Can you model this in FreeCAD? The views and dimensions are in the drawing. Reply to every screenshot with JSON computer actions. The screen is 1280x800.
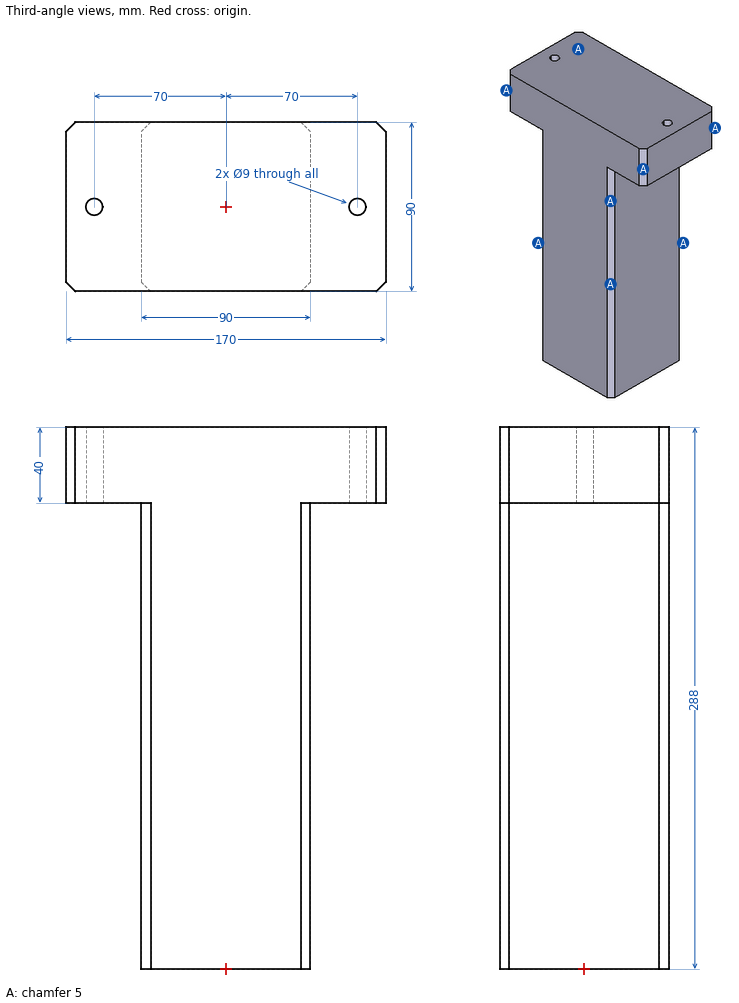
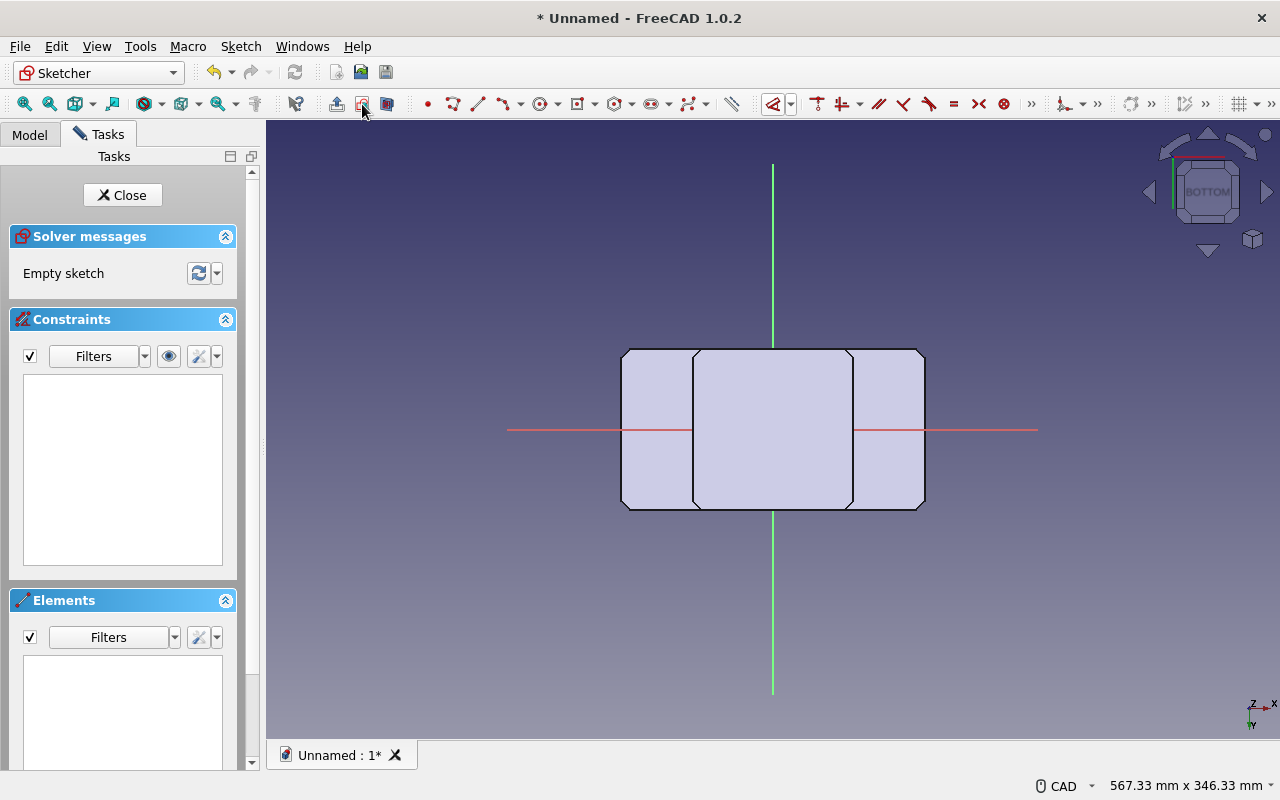
{"action": "scroll", "coordinate": [829, 430], "scroll_direction": "up", "scroll_amount": 4}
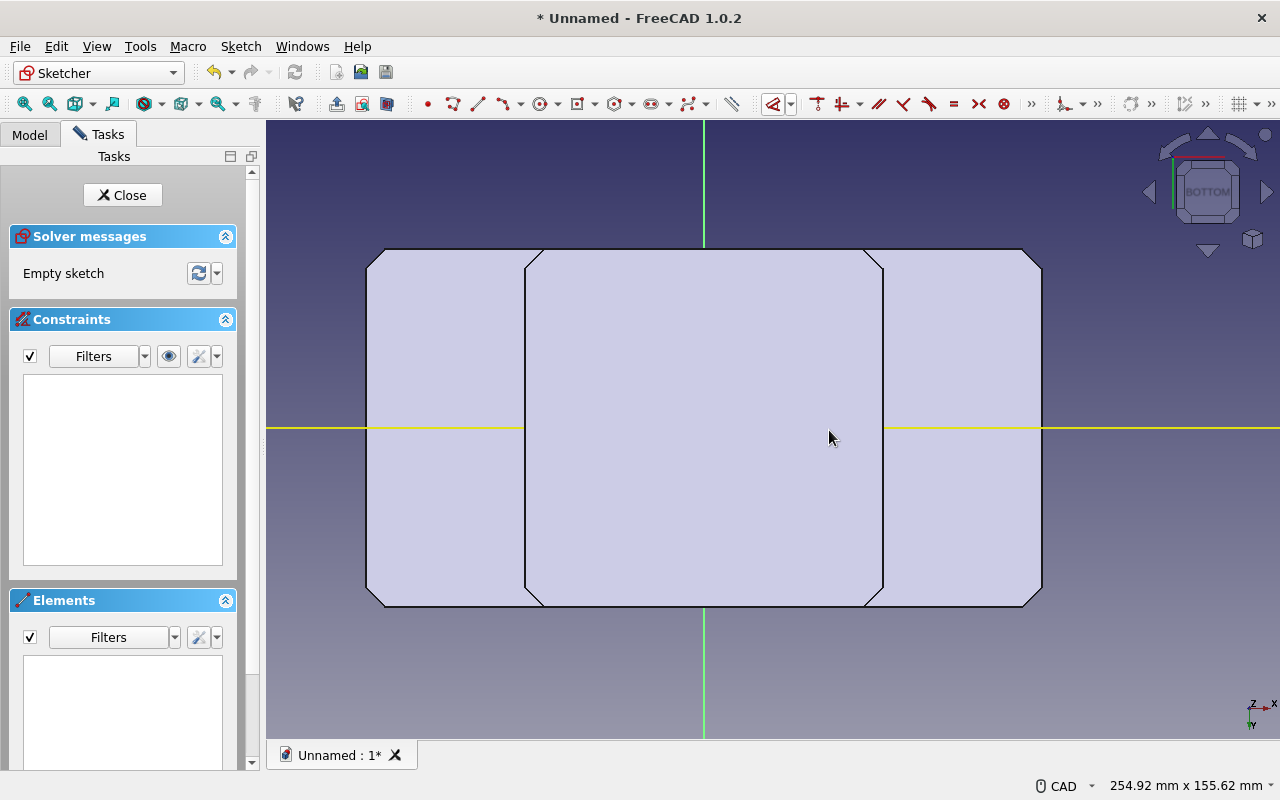
{"action": "left_click", "coordinate": [540, 104]}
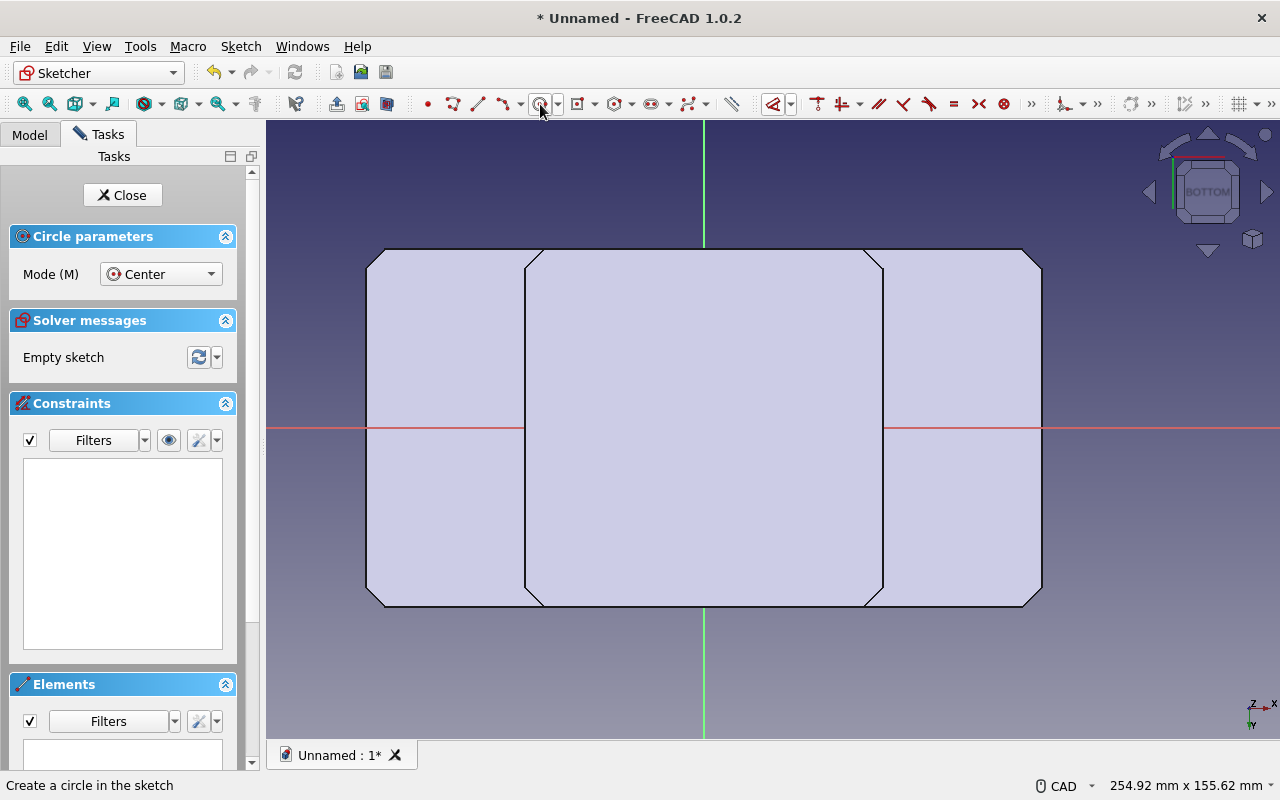
{"action": "scroll", "coordinate": [982, 428], "scroll_direction": "up", "scroll_amount": 2}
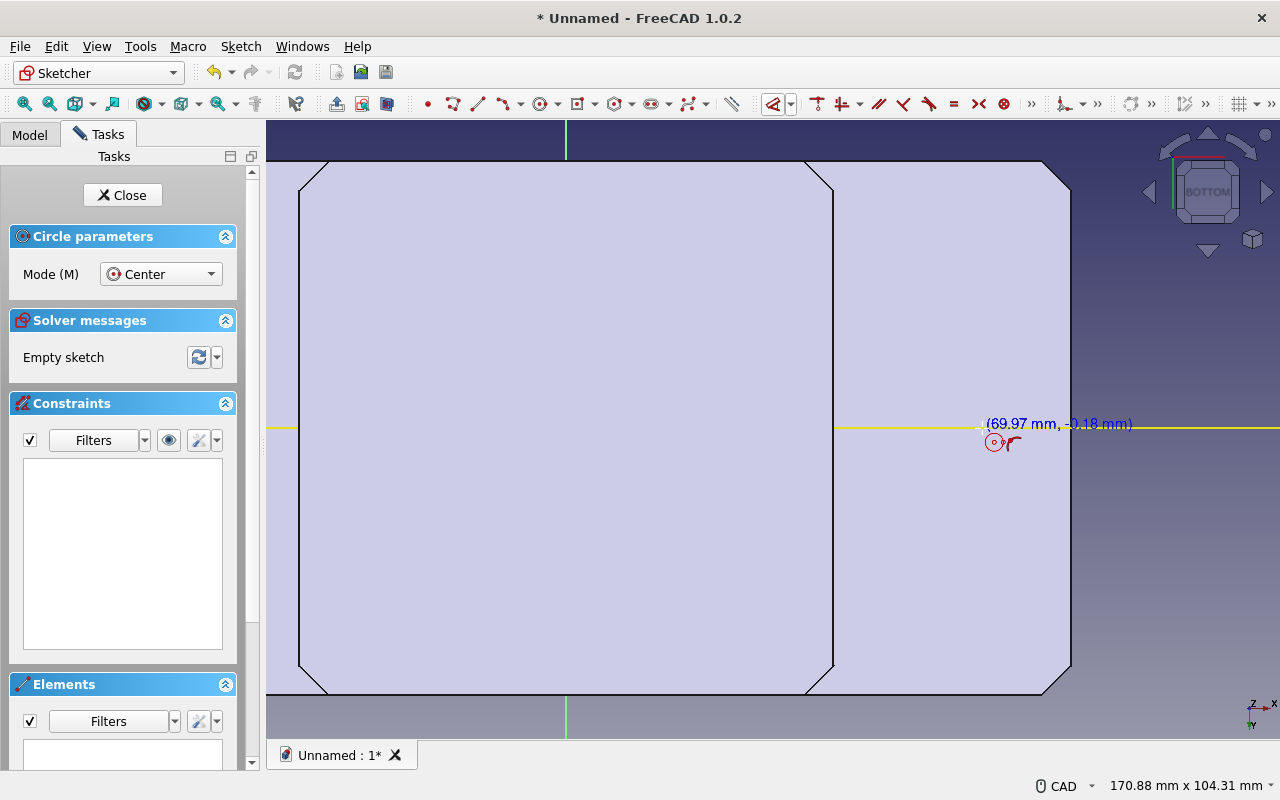
{"action": "left_click", "coordinate": [982, 428]}
{"action": "left_click", "coordinate": [1001, 409]}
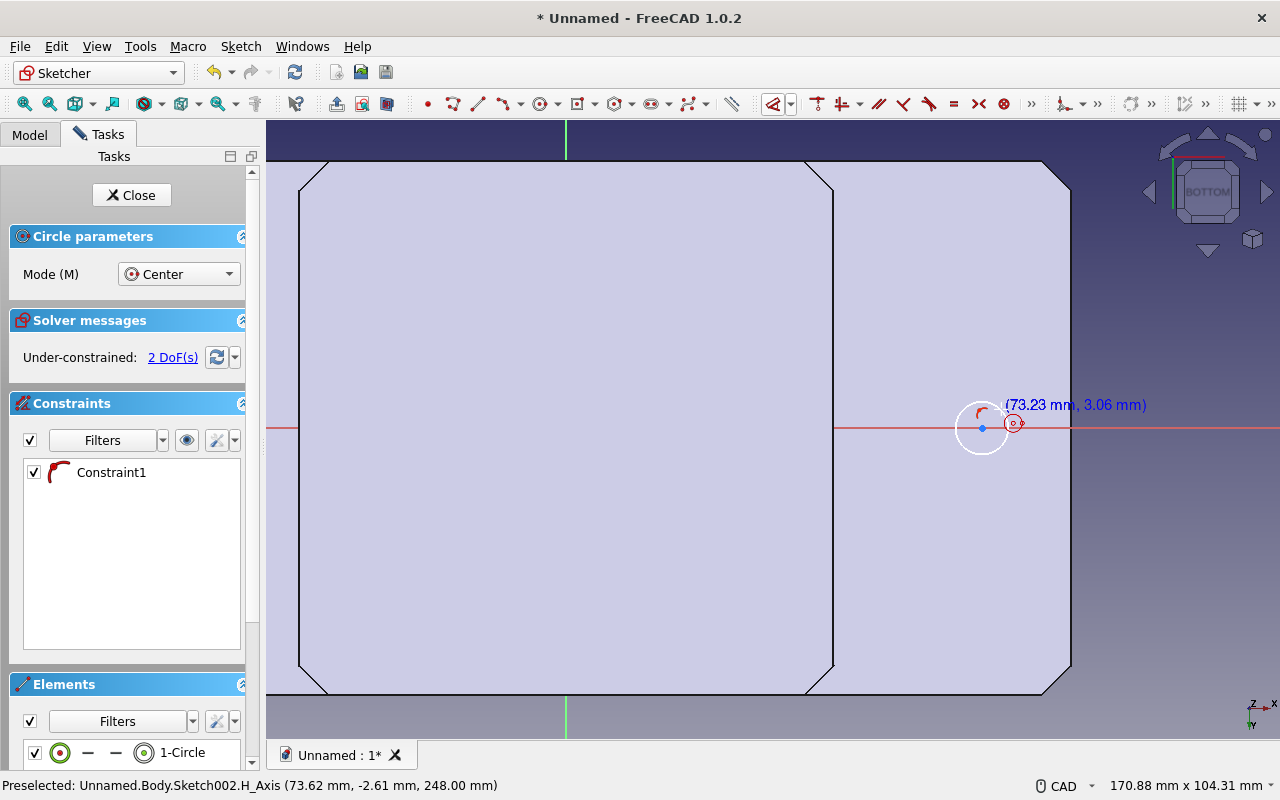
{"action": "scroll", "coordinate": [985, 432], "scroll_direction": "down", "scroll_amount": 2}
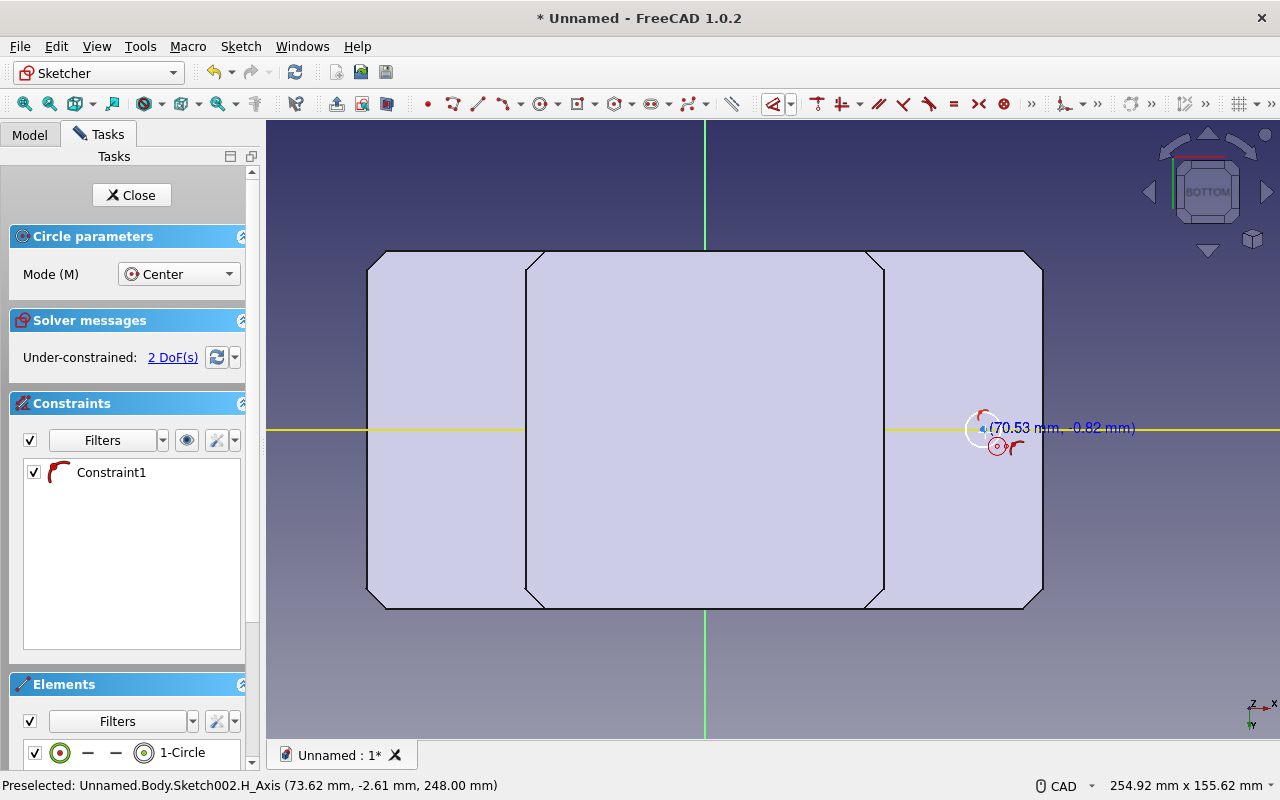
{"action": "scroll", "coordinate": [426, 430], "scroll_direction": "up", "scroll_amount": 2}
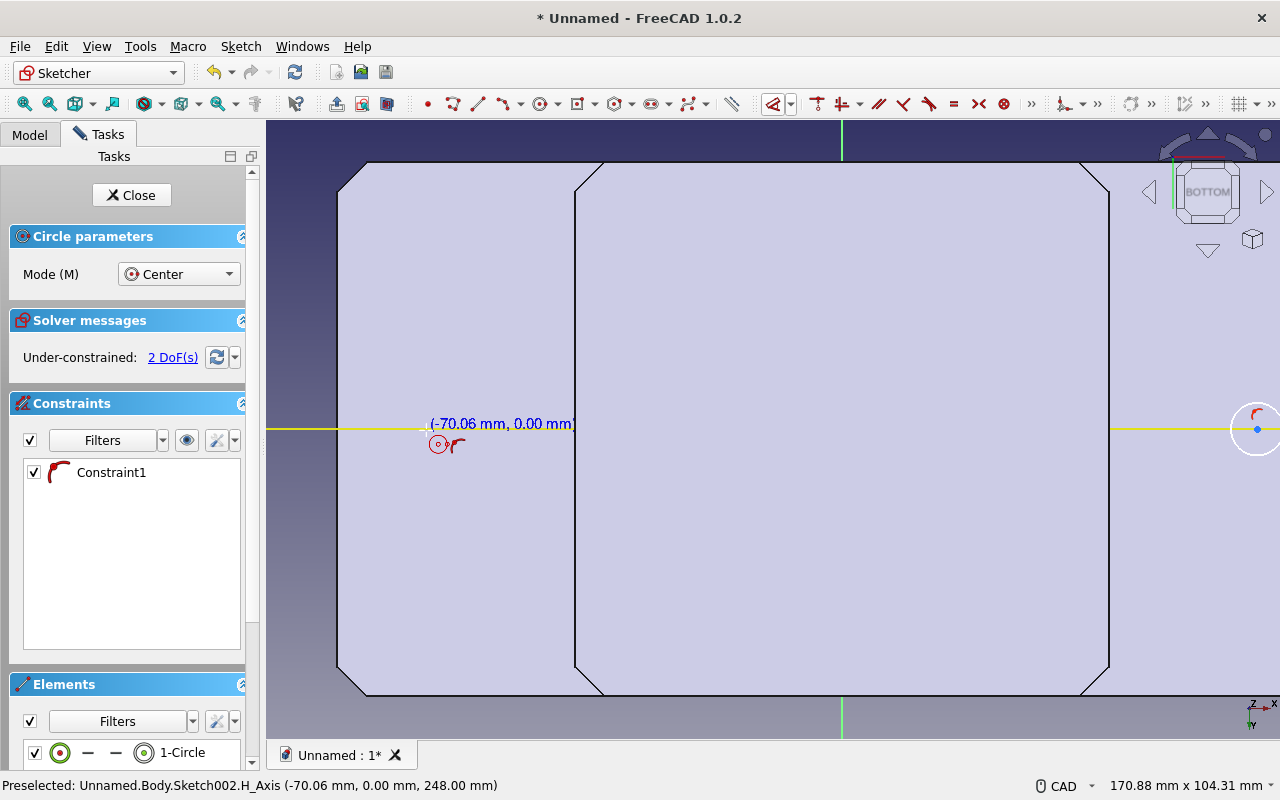
{"action": "left_click", "coordinate": [426, 429]}
{"action": "left_click", "coordinate": [445, 410]}
{"action": "key", "text": "Escape"}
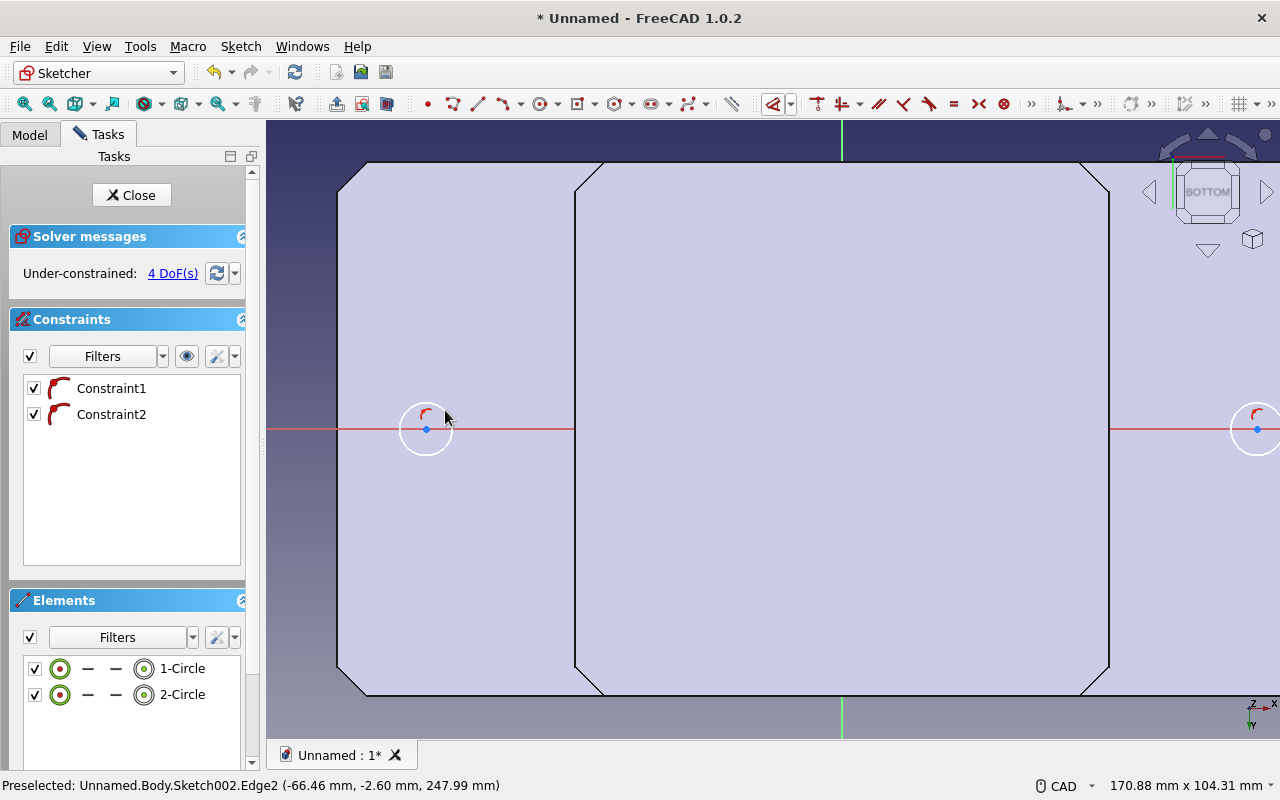
{"action": "scroll", "coordinate": [426, 430], "scroll_direction": "down", "scroll_amount": 2}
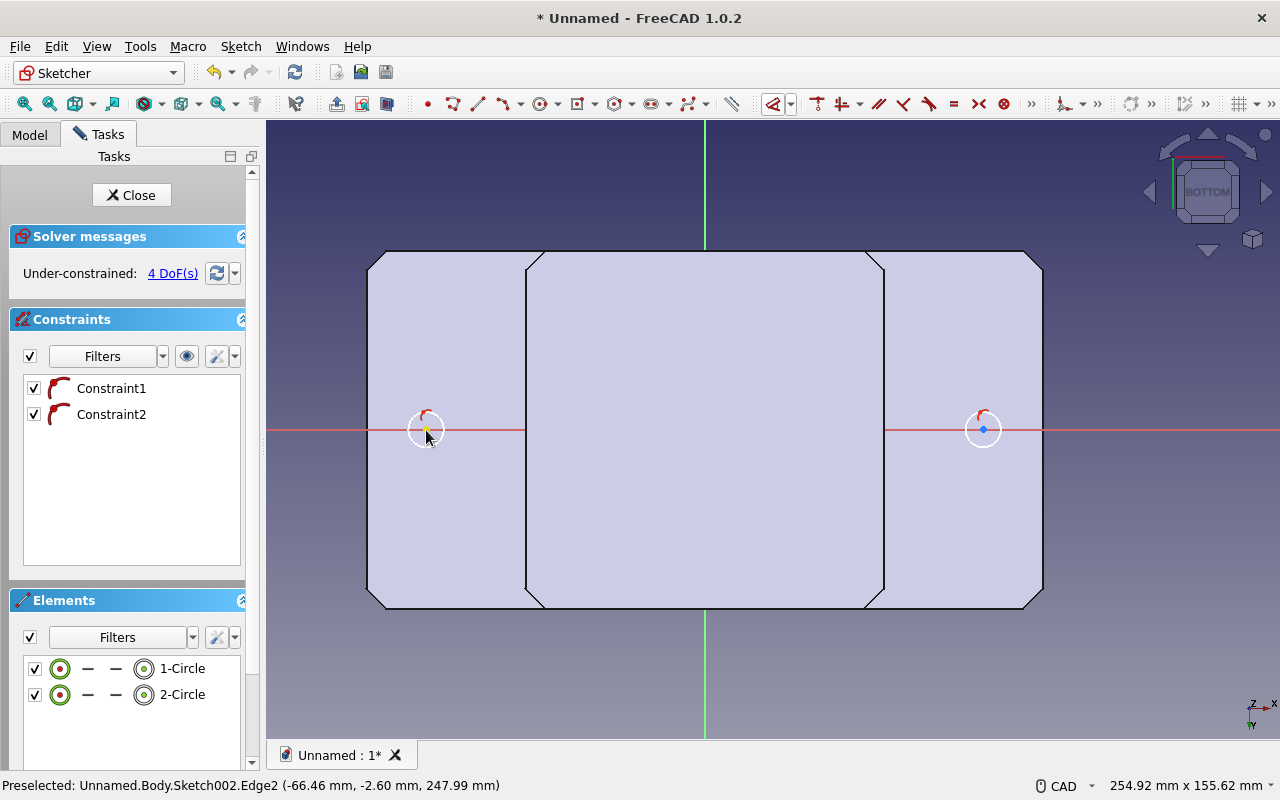
{"action": "left_click", "coordinate": [996, 417]}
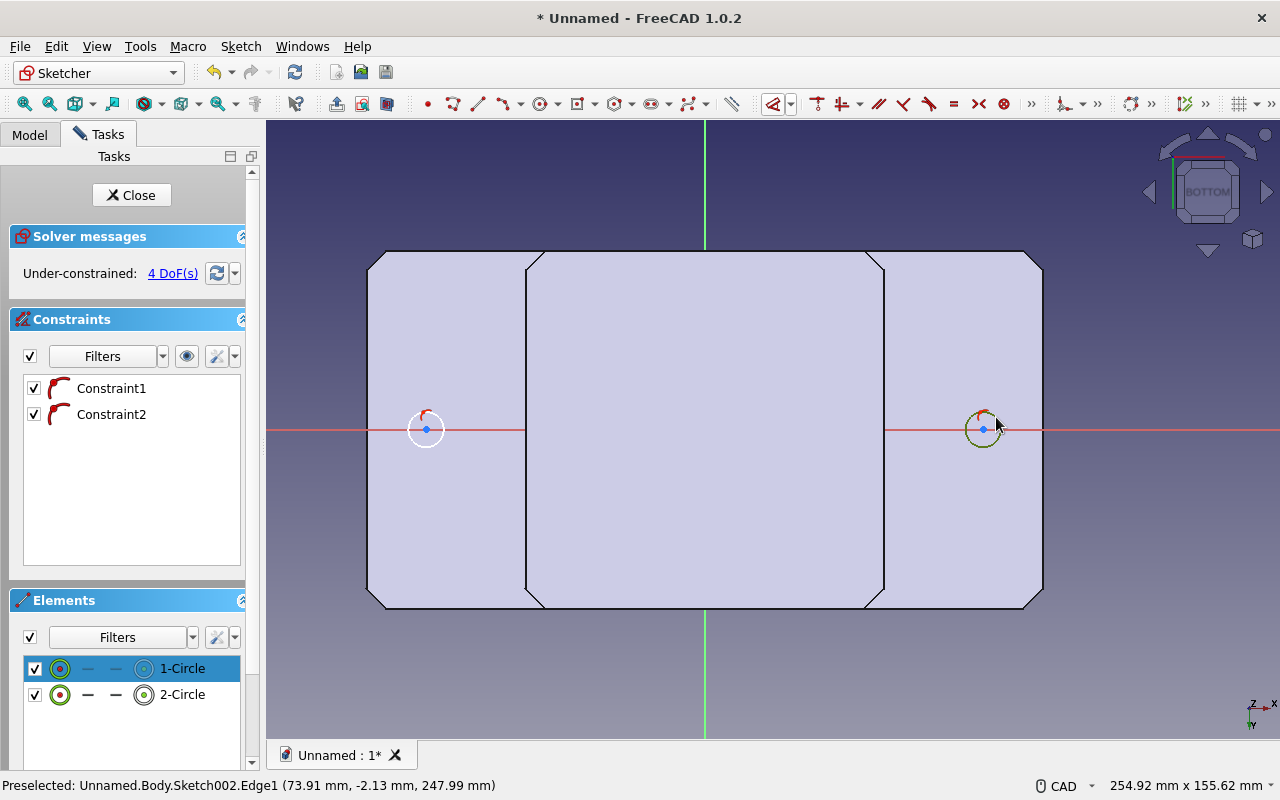
{"action": "left_click", "coordinate": [438, 417]}